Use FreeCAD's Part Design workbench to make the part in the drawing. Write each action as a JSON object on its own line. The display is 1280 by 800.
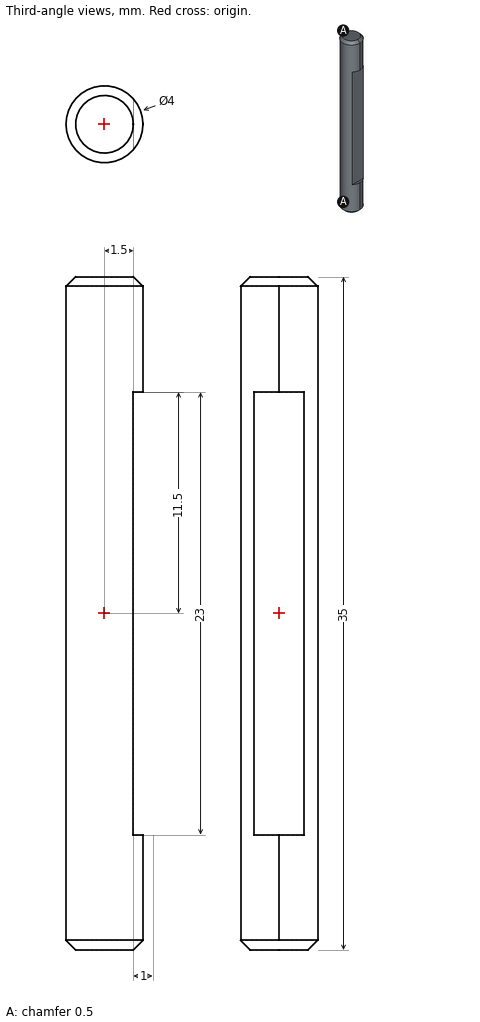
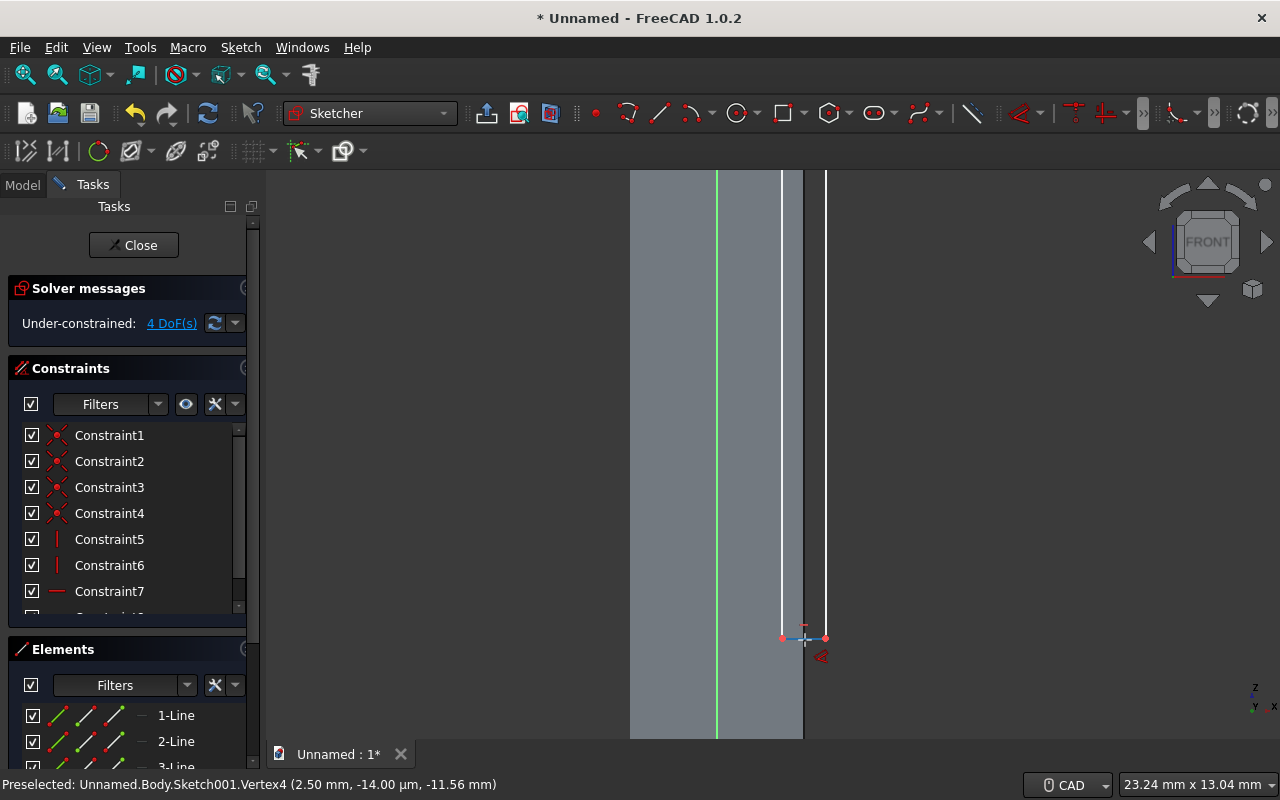
{"action": "left_click", "coordinate": [804, 639]}
{"action": "left_click", "coordinate": [804, 673]}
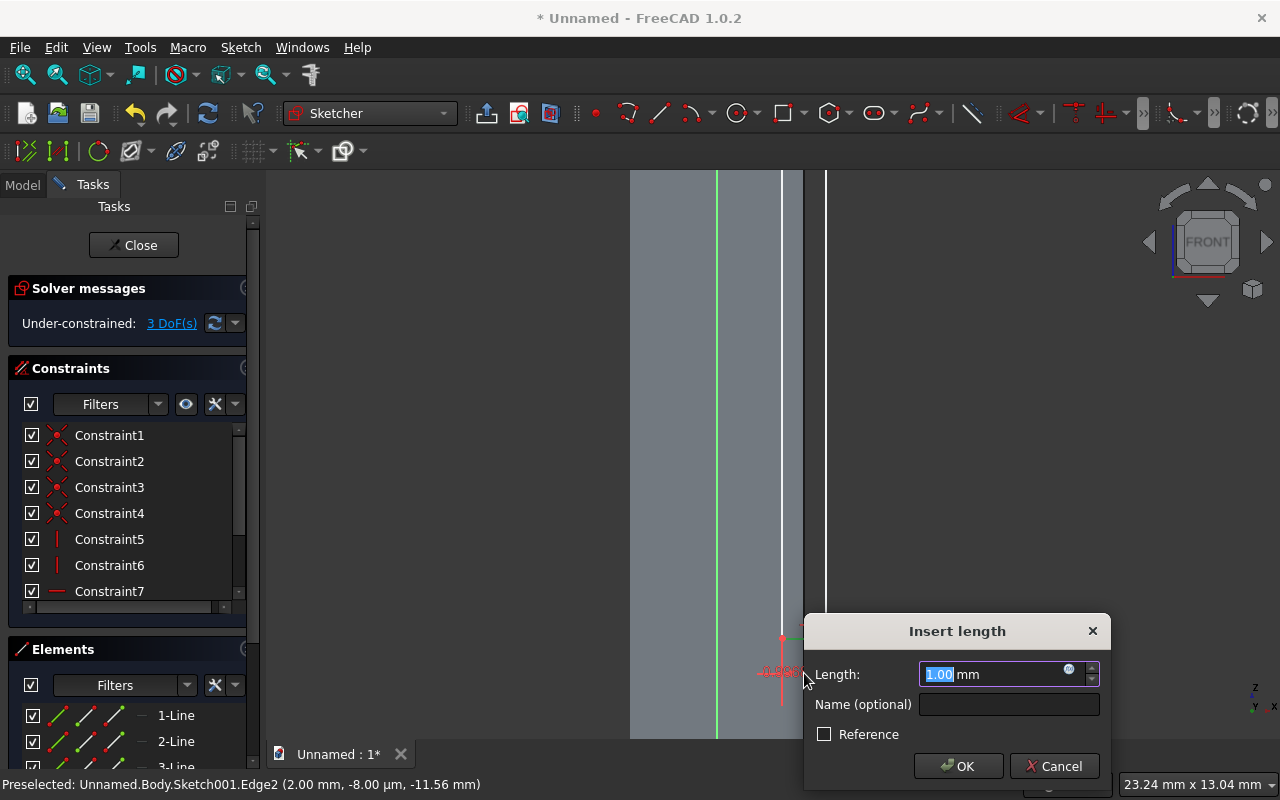
{"action": "type", "text": "1"}
{"action": "key", "text": "Return"}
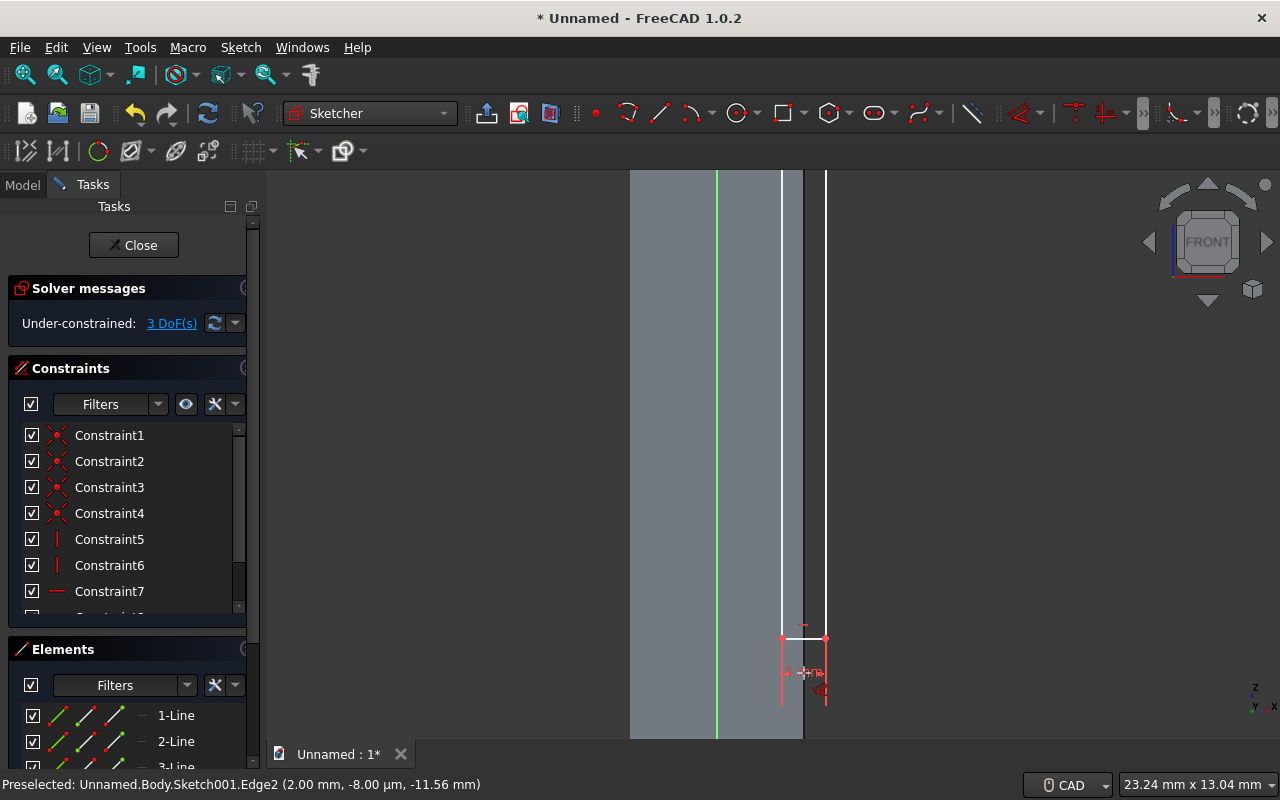
{"action": "left_click", "coordinate": [782, 338]}
{"action": "left_click", "coordinate": [748, 418]}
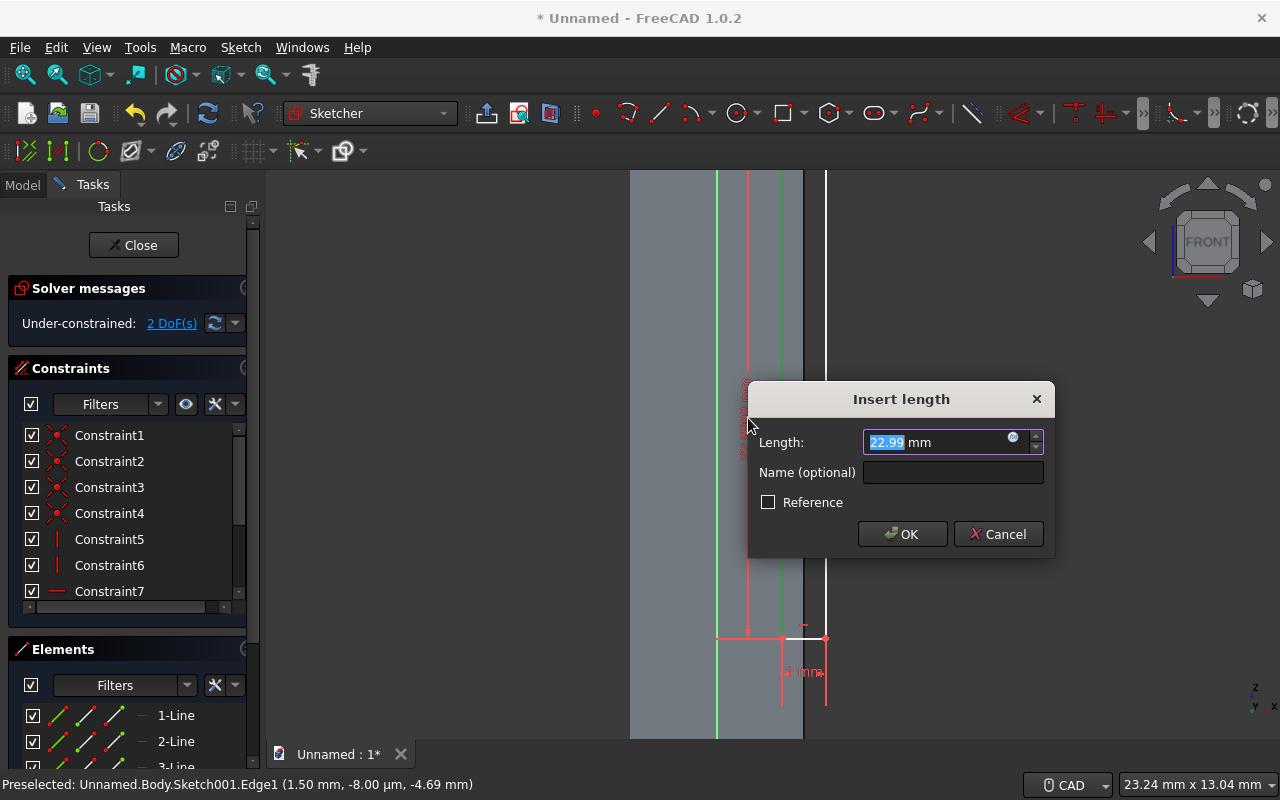
{"action": "type", "text": "23"}
{"action": "key", "text": "Return"}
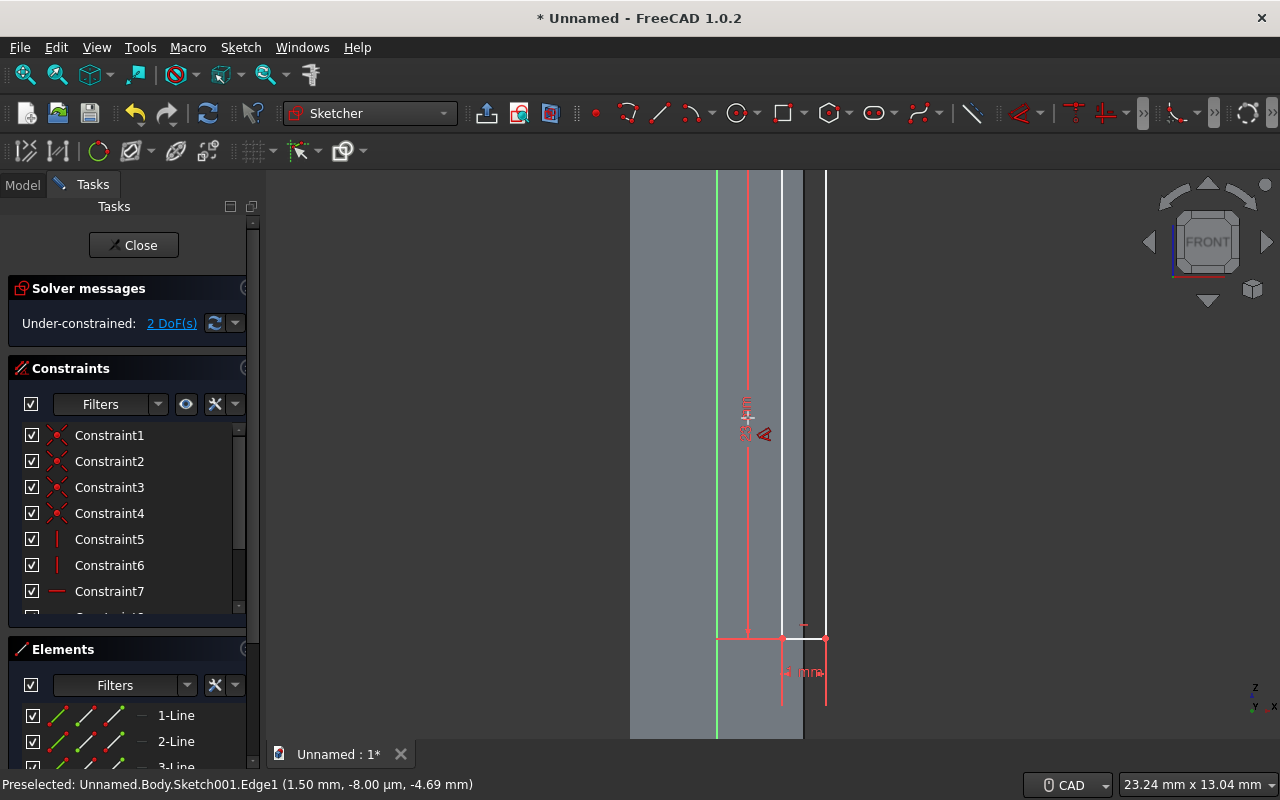
{"action": "scroll", "coordinate": [666, 641], "scroll_direction": "down", "scroll_amount": 5}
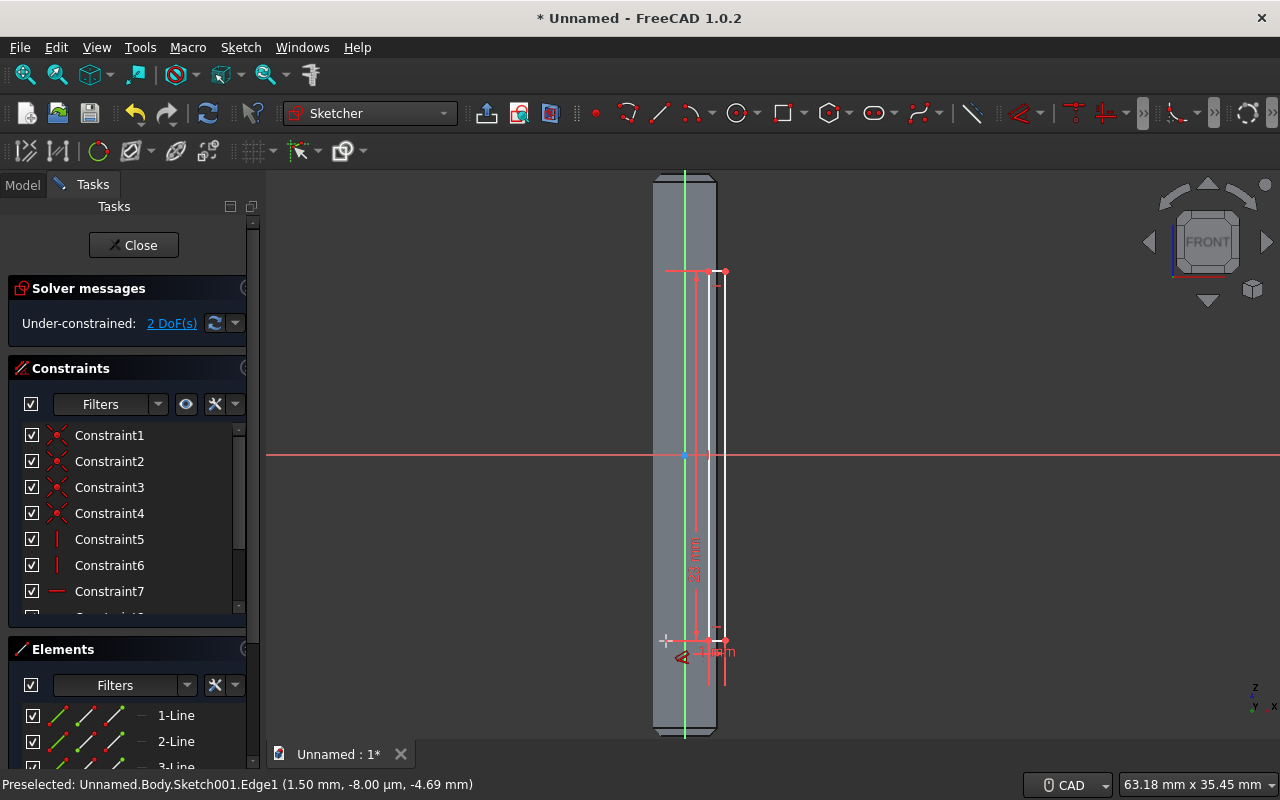
{"action": "scroll", "coordinate": [709, 271], "scroll_direction": "up", "scroll_amount": 3}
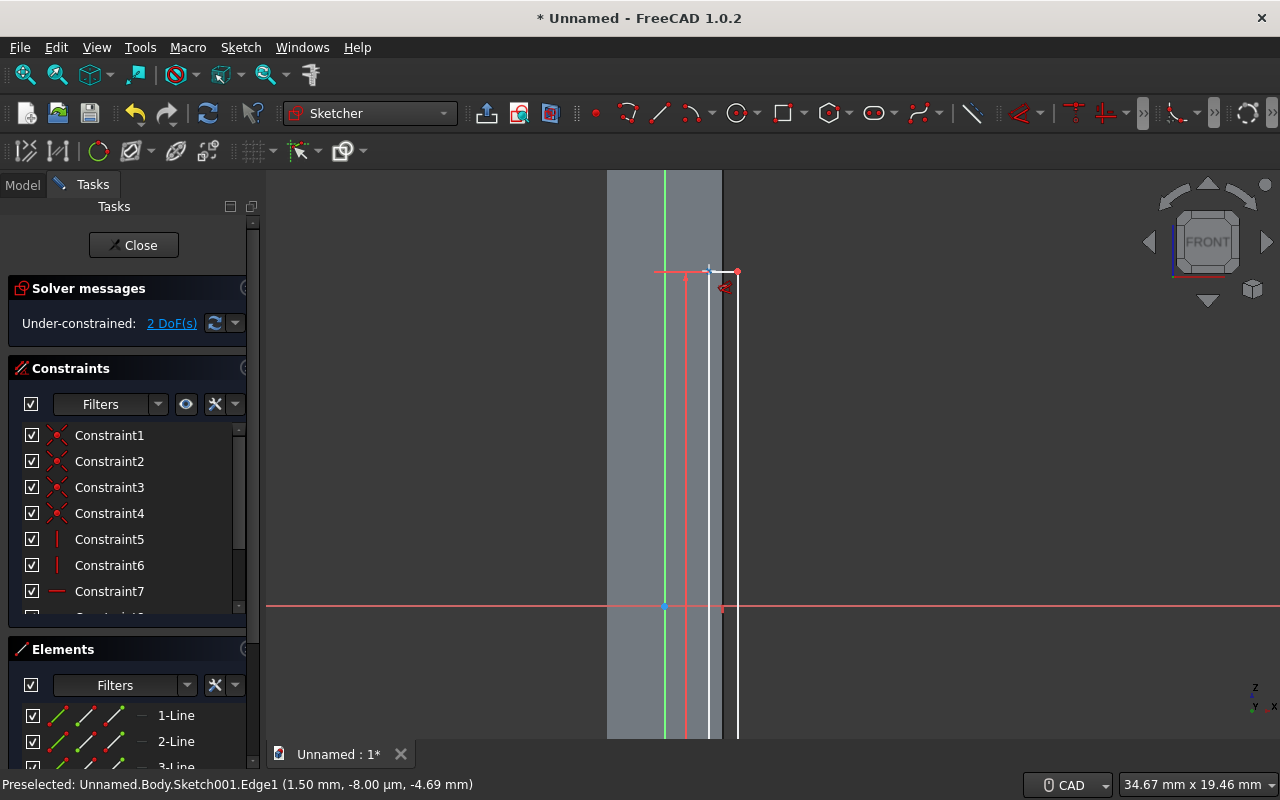
{"action": "left_click", "coordinate": [709, 272]}
{"action": "left_click", "coordinate": [687, 238]}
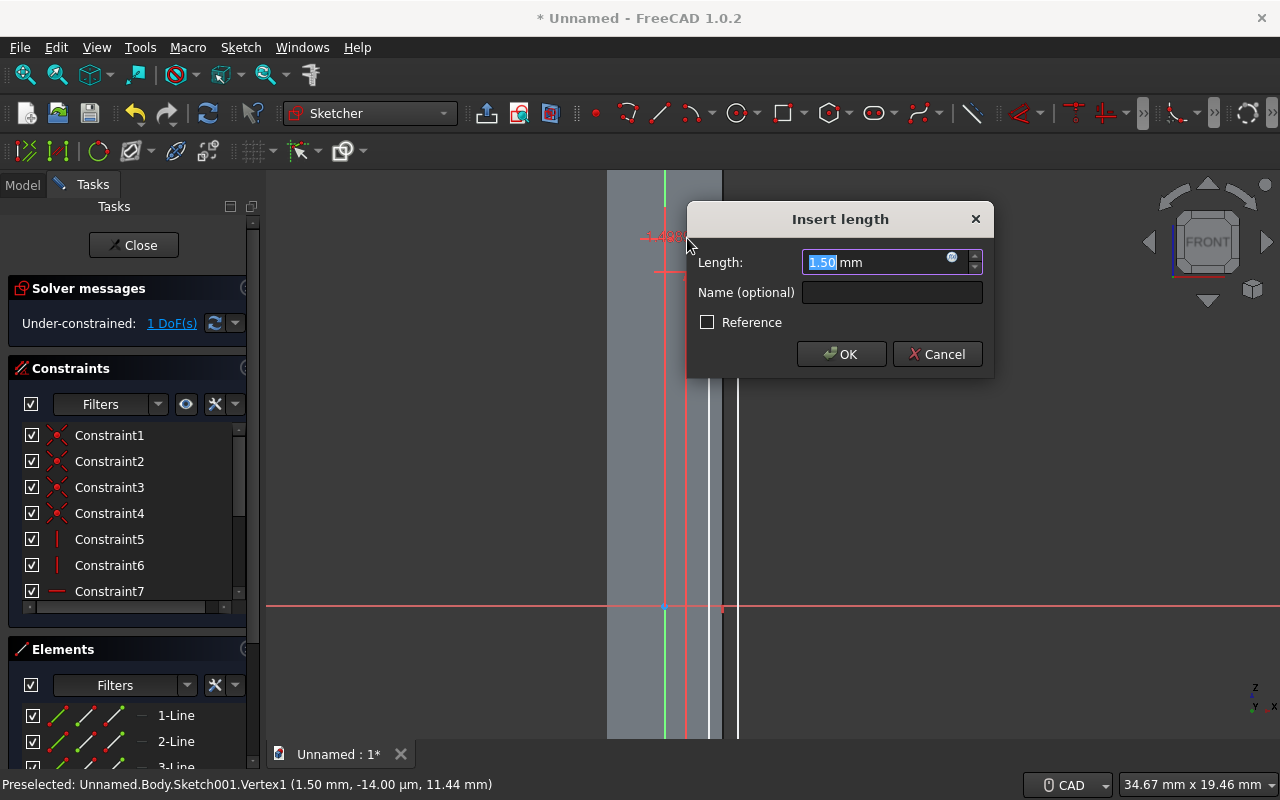
{"action": "type", "text": "1.5"}
{"action": "key", "text": "Return"}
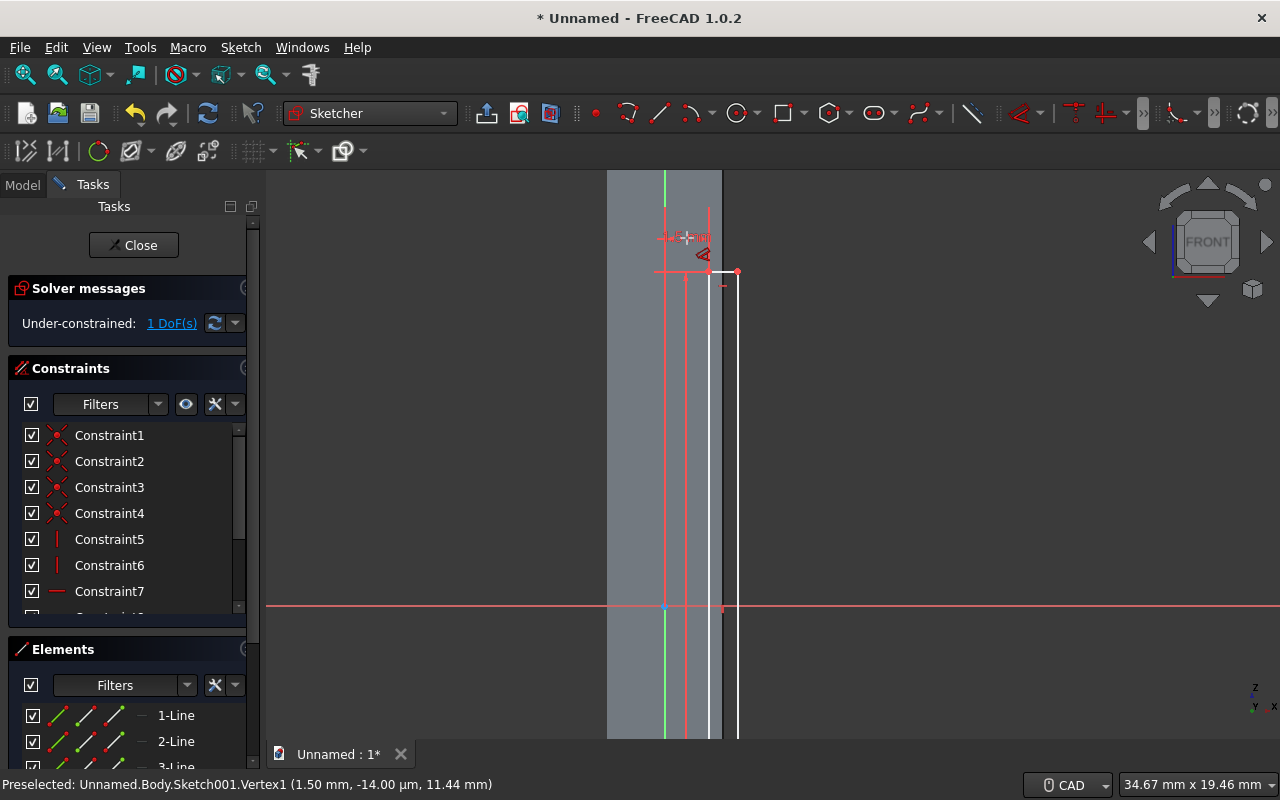
{"action": "left_click", "coordinate": [709, 272]}
{"action": "left_click", "coordinate": [631, 439]}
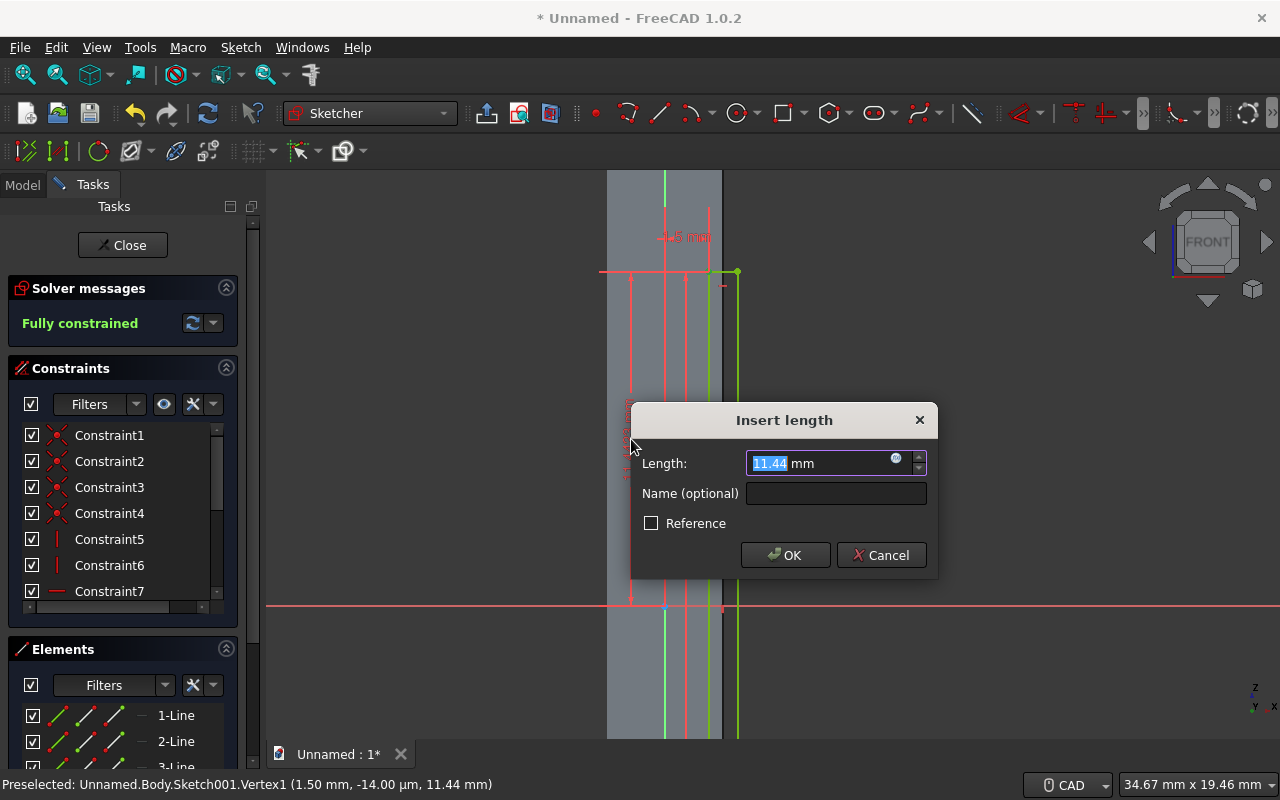
{"action": "type", "text": "11.5"}
{"action": "key", "text": "Return"}
{"action": "key", "text": "Escape"}